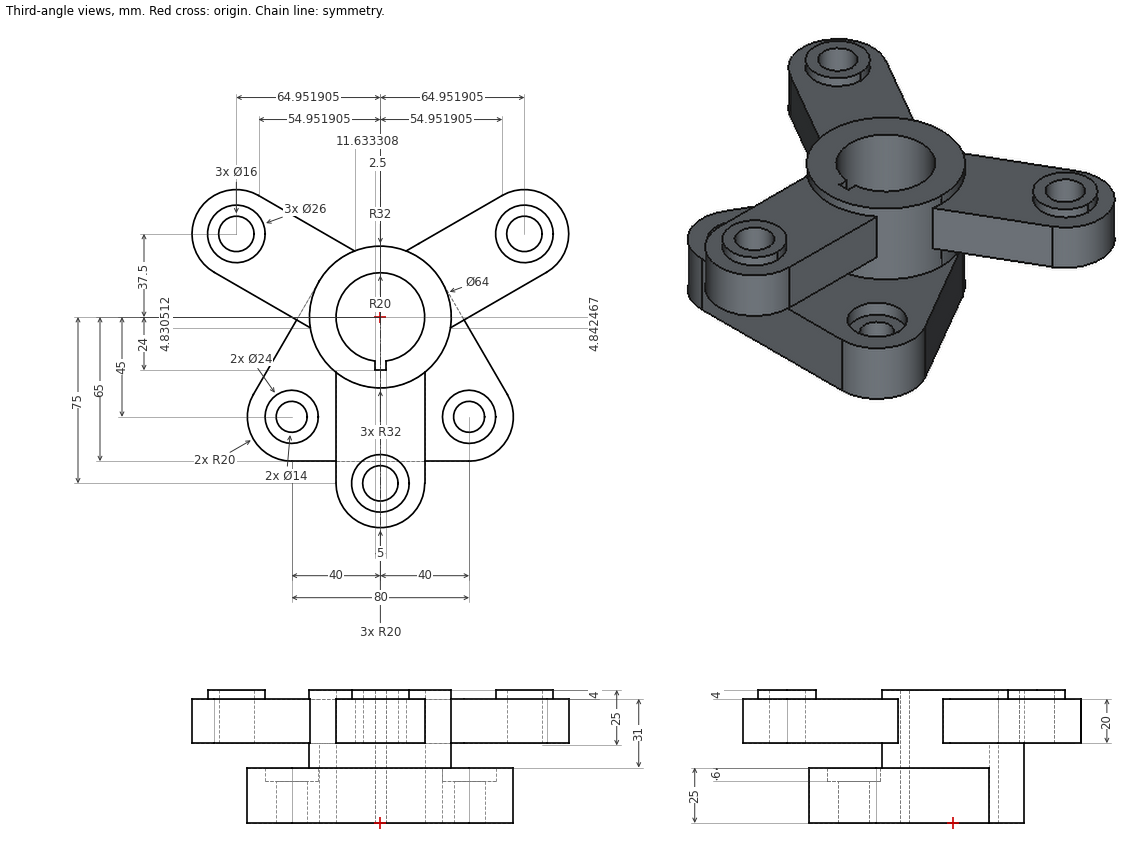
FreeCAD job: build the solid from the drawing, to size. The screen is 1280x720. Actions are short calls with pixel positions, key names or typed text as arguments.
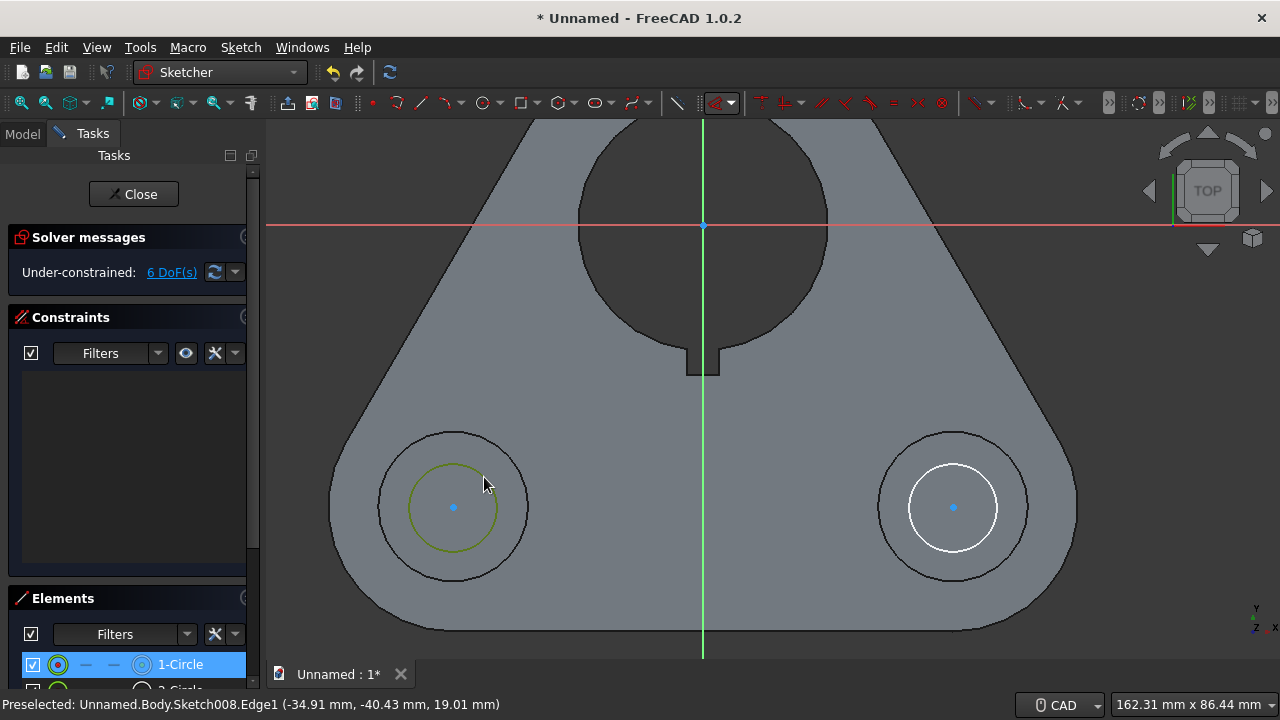
click(984, 477)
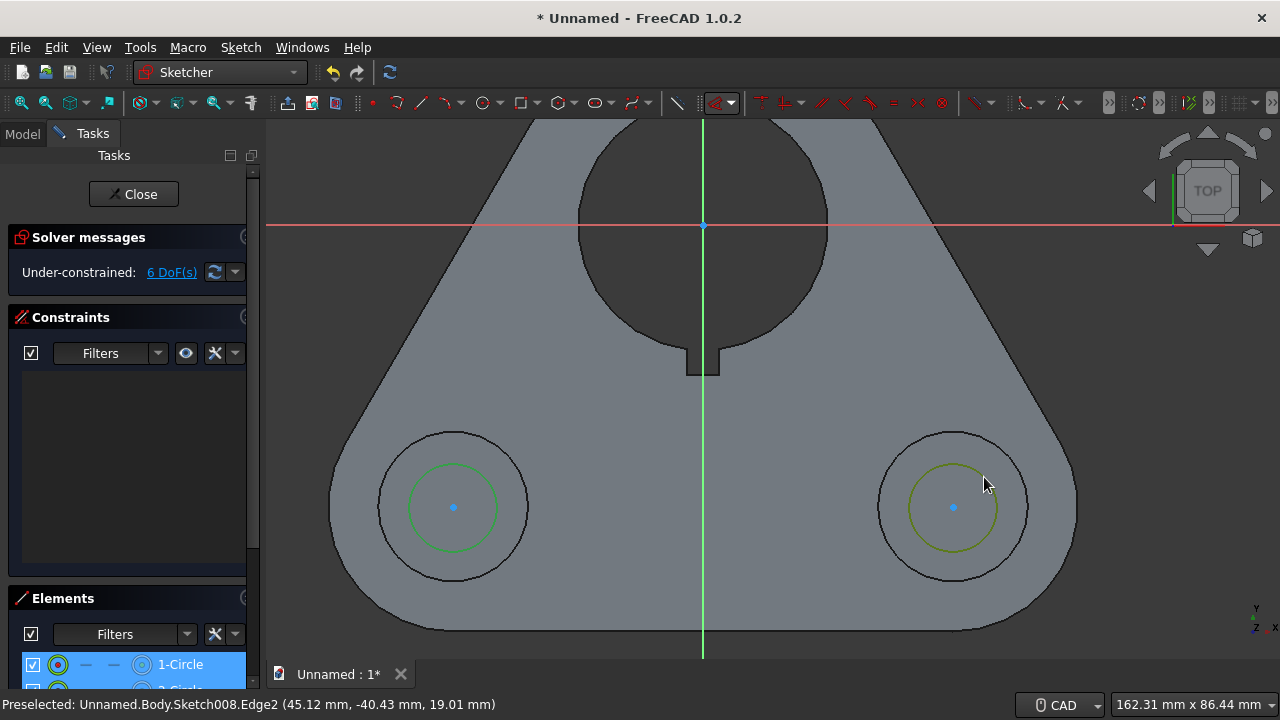
key(e)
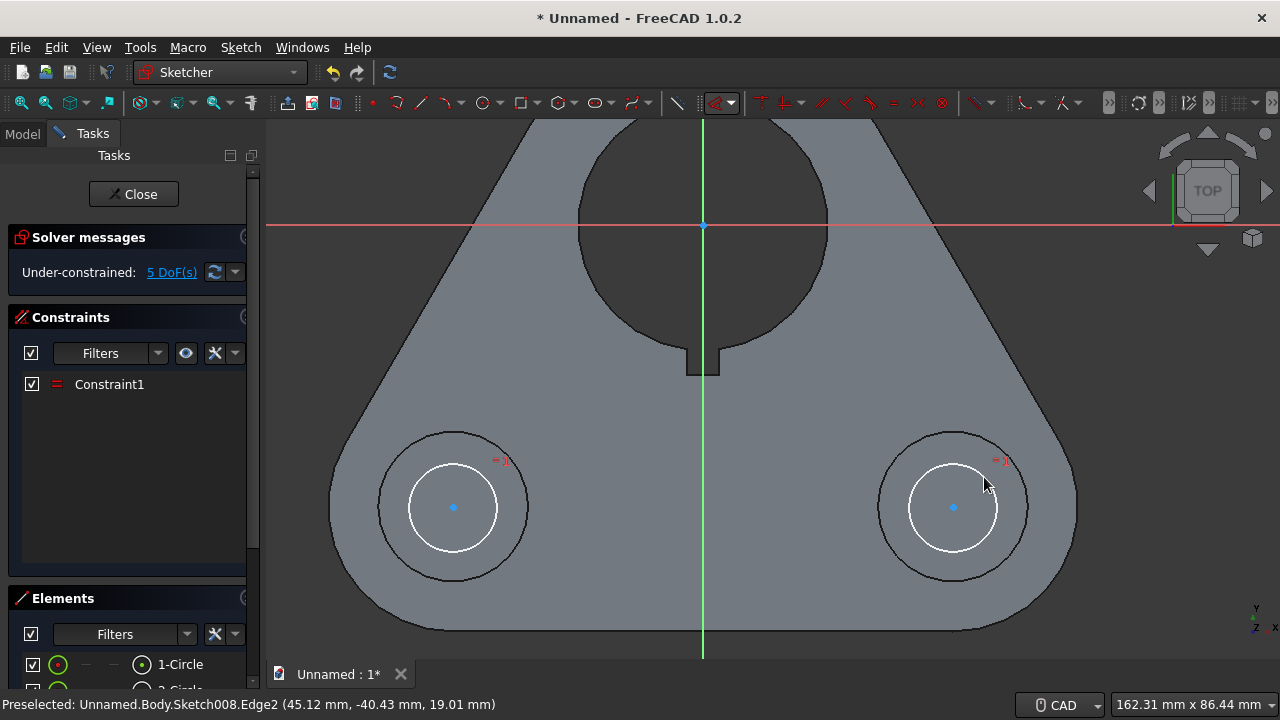
click(453, 508)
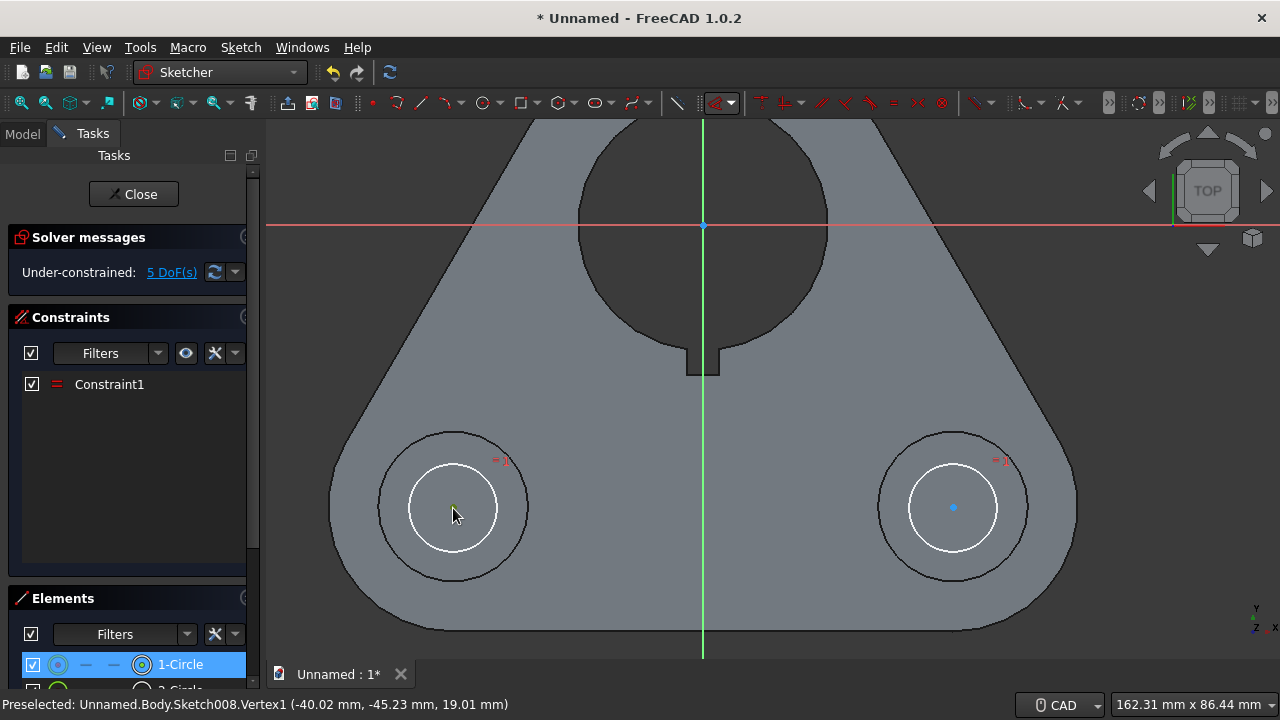
click(953, 508)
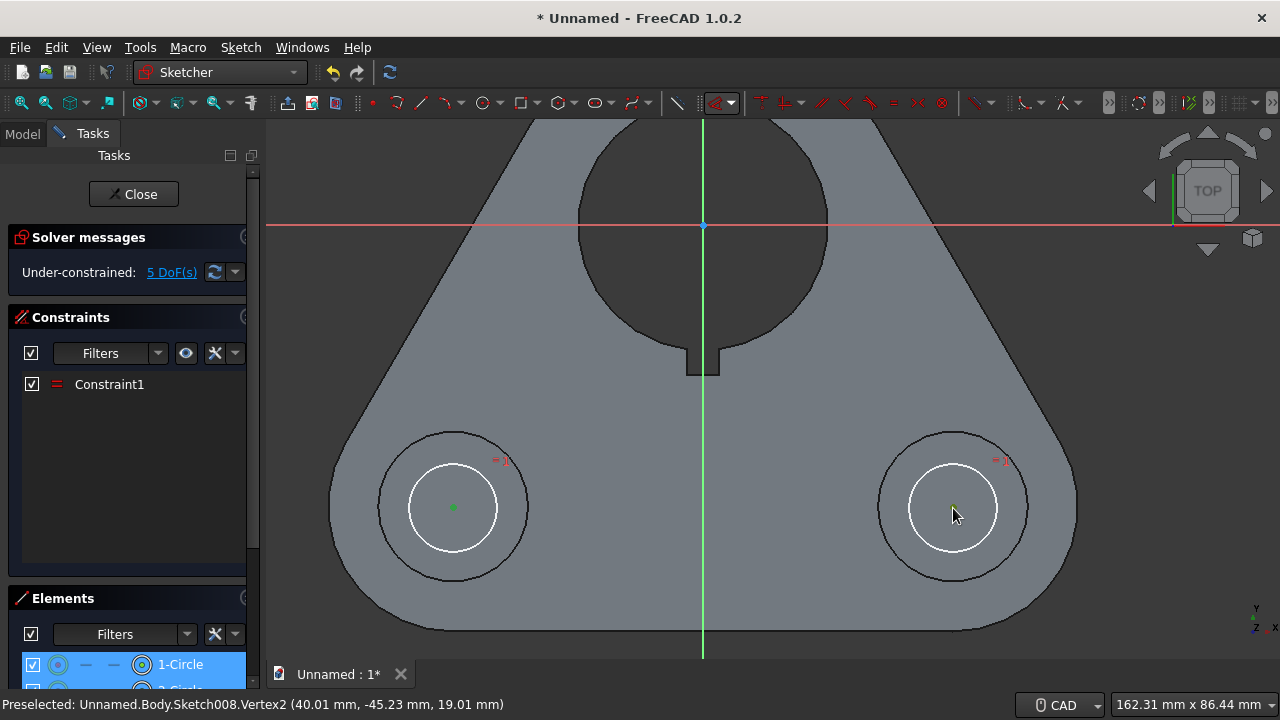
key(h)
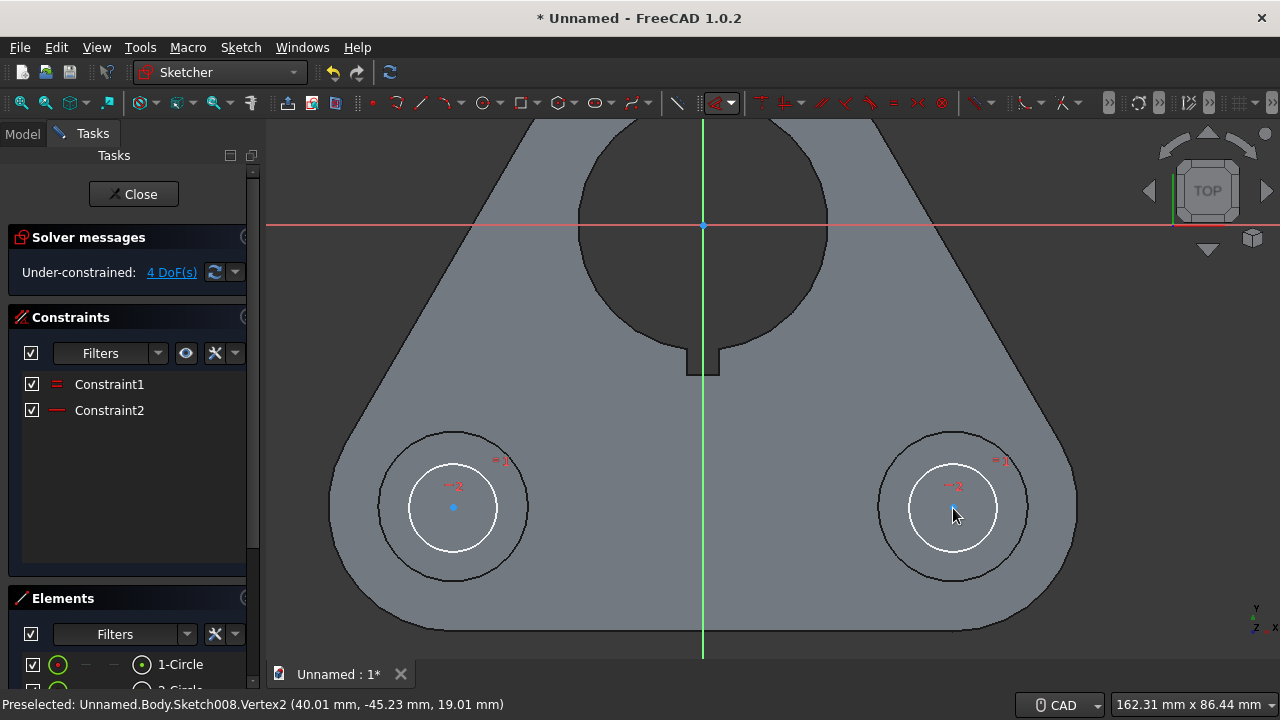
click(484, 477)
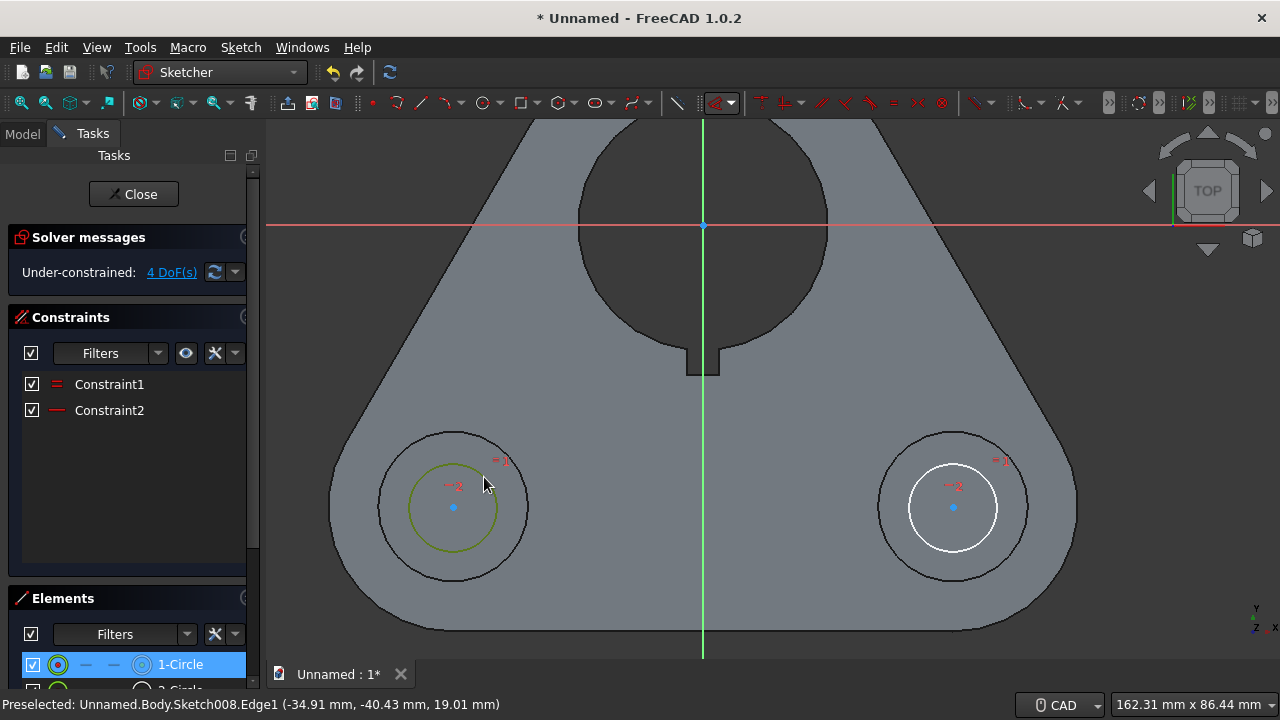
key(k)
key(o)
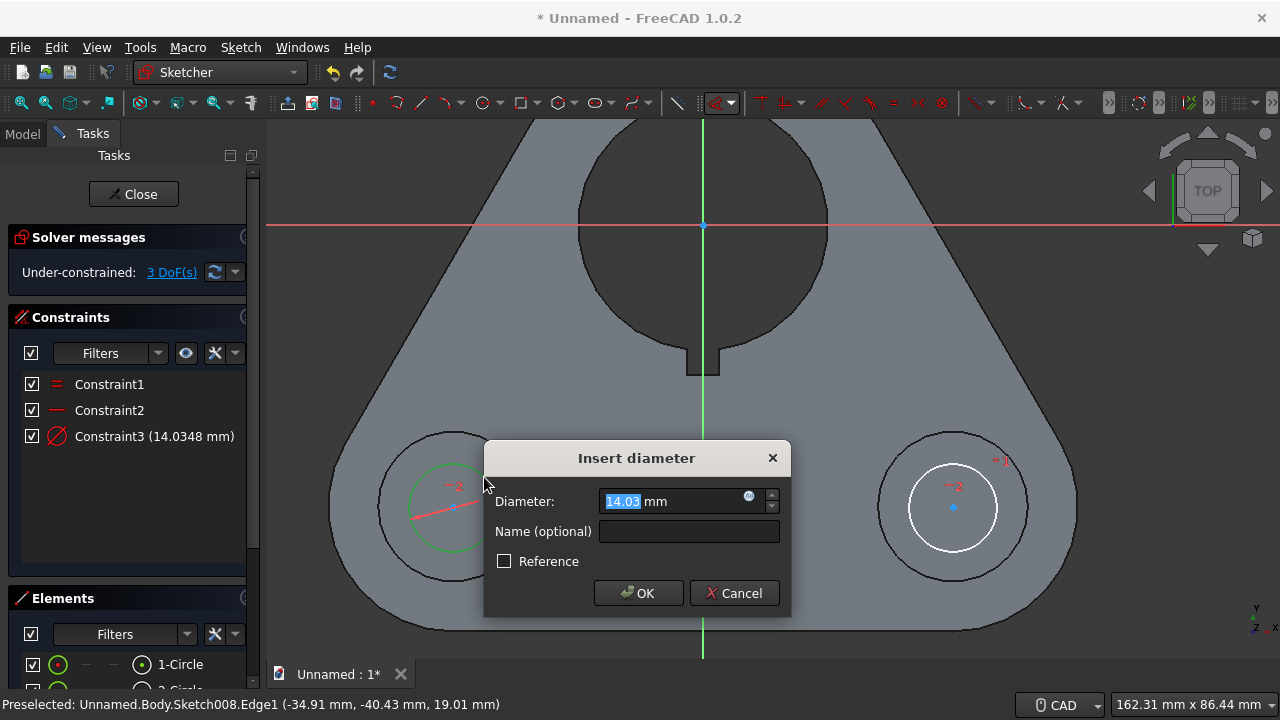
text(14)
key(Return)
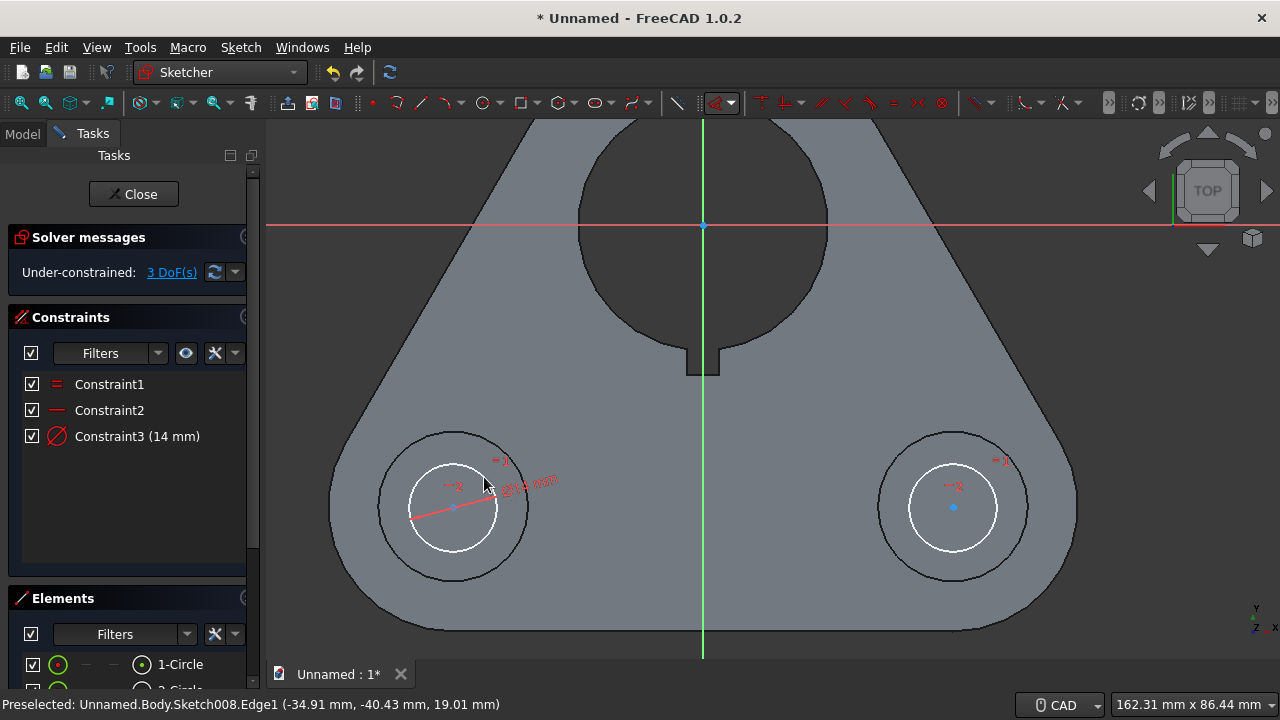
click(453, 508)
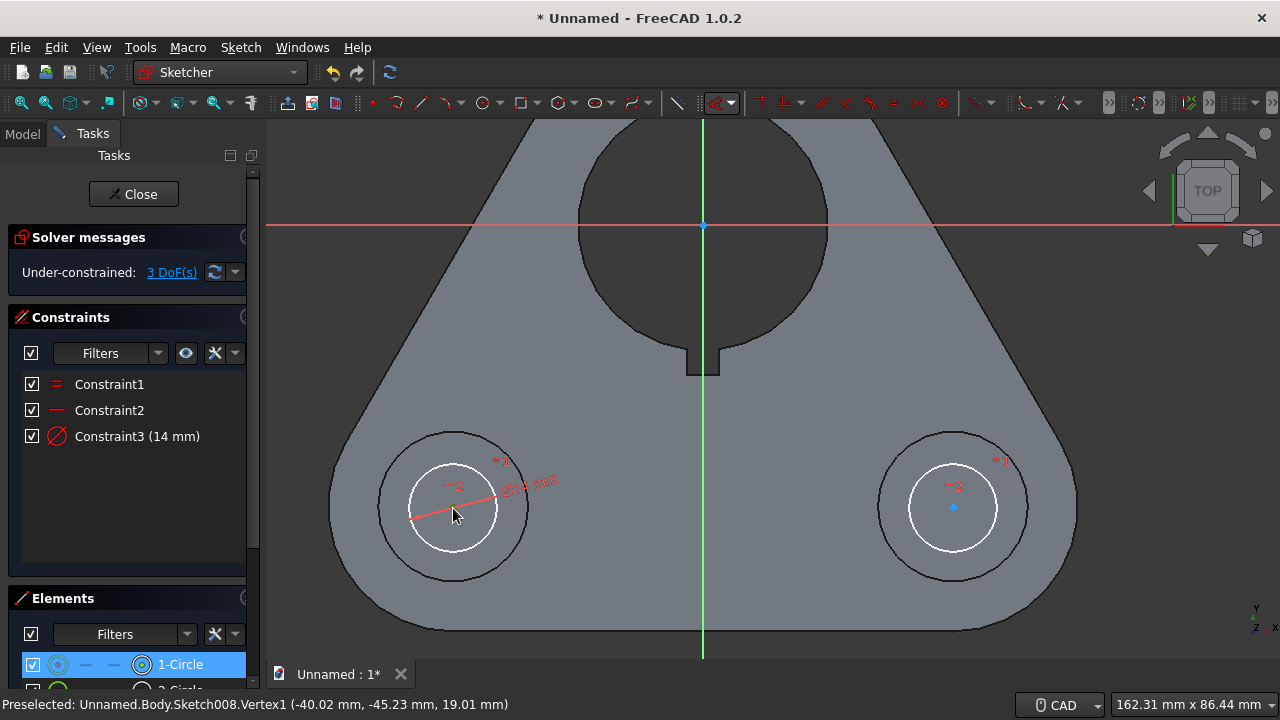
key(l)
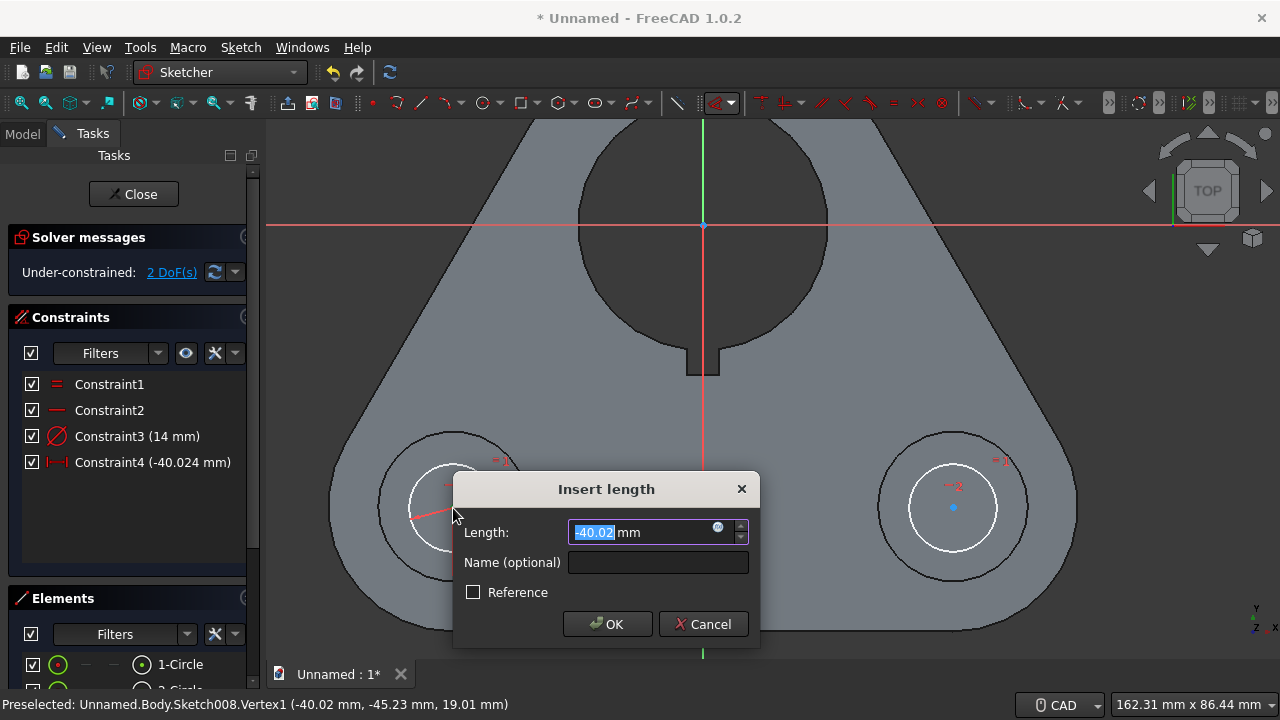
text(-40)
key(Return)